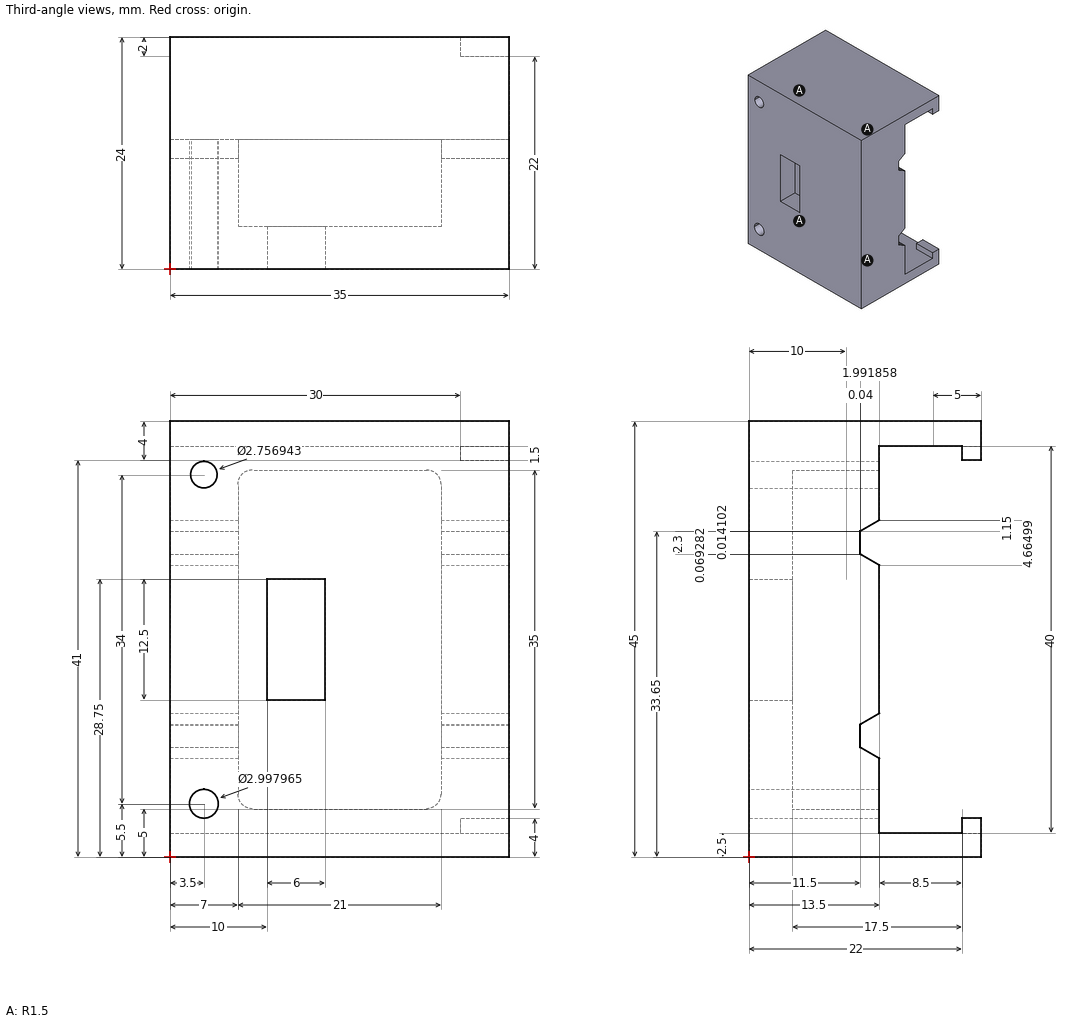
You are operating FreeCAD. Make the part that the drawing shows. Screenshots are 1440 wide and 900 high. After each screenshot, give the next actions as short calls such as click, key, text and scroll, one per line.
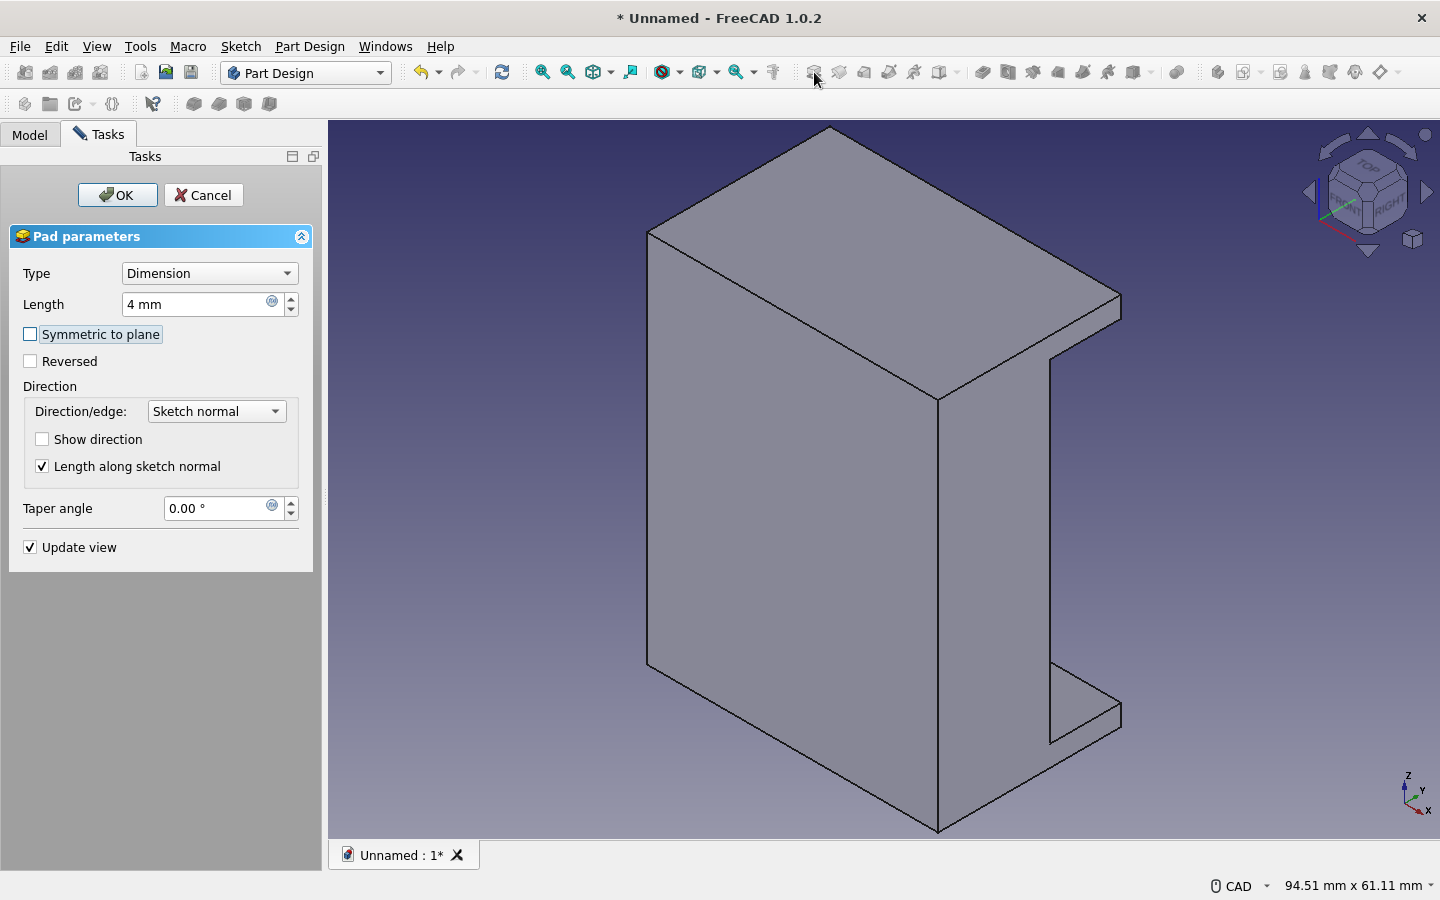
click(31, 361)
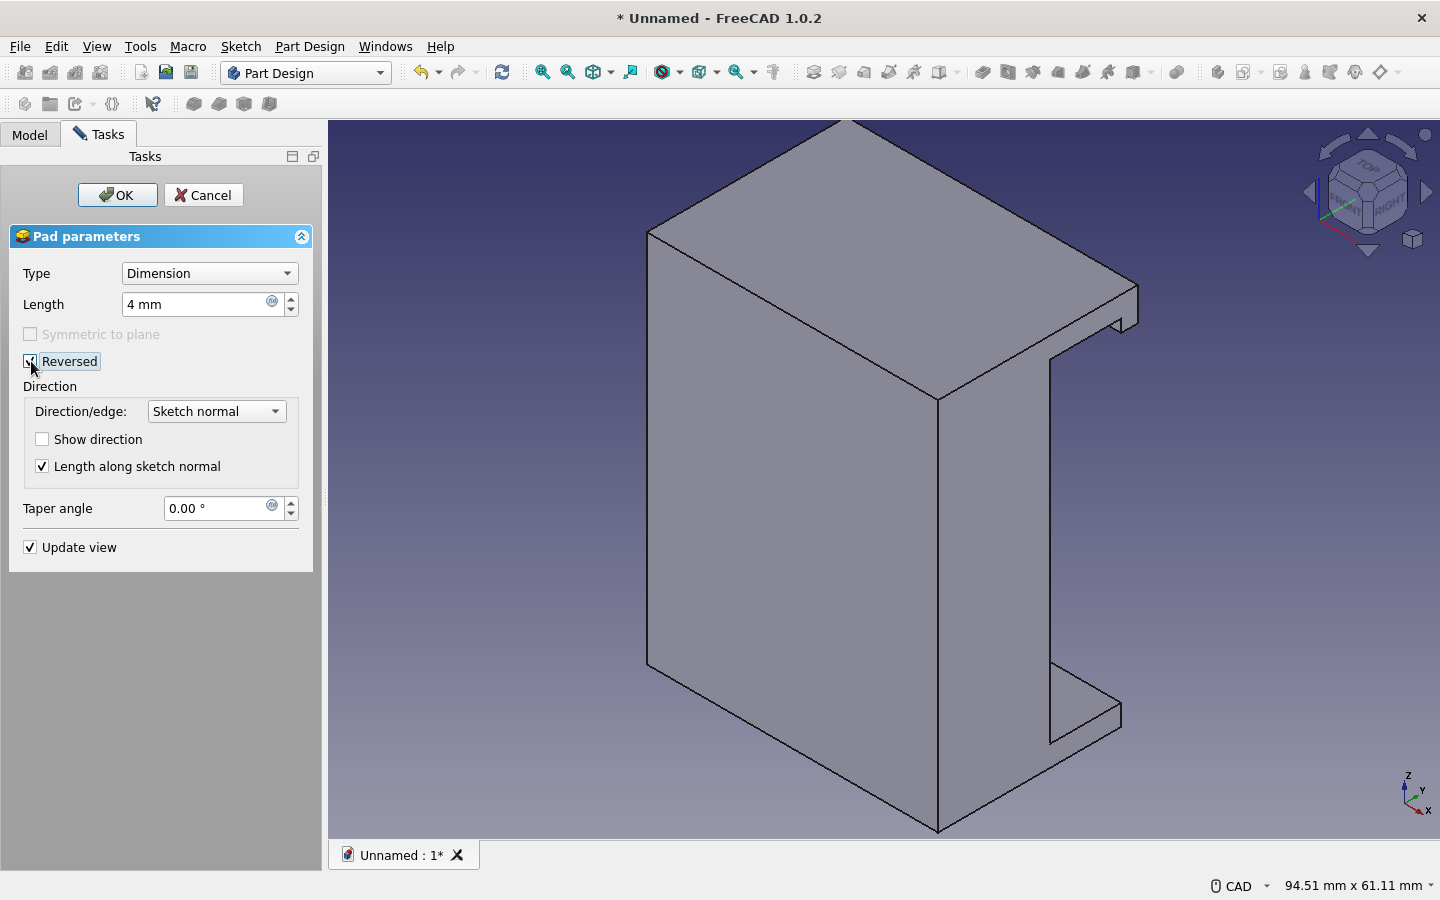
click(118, 195)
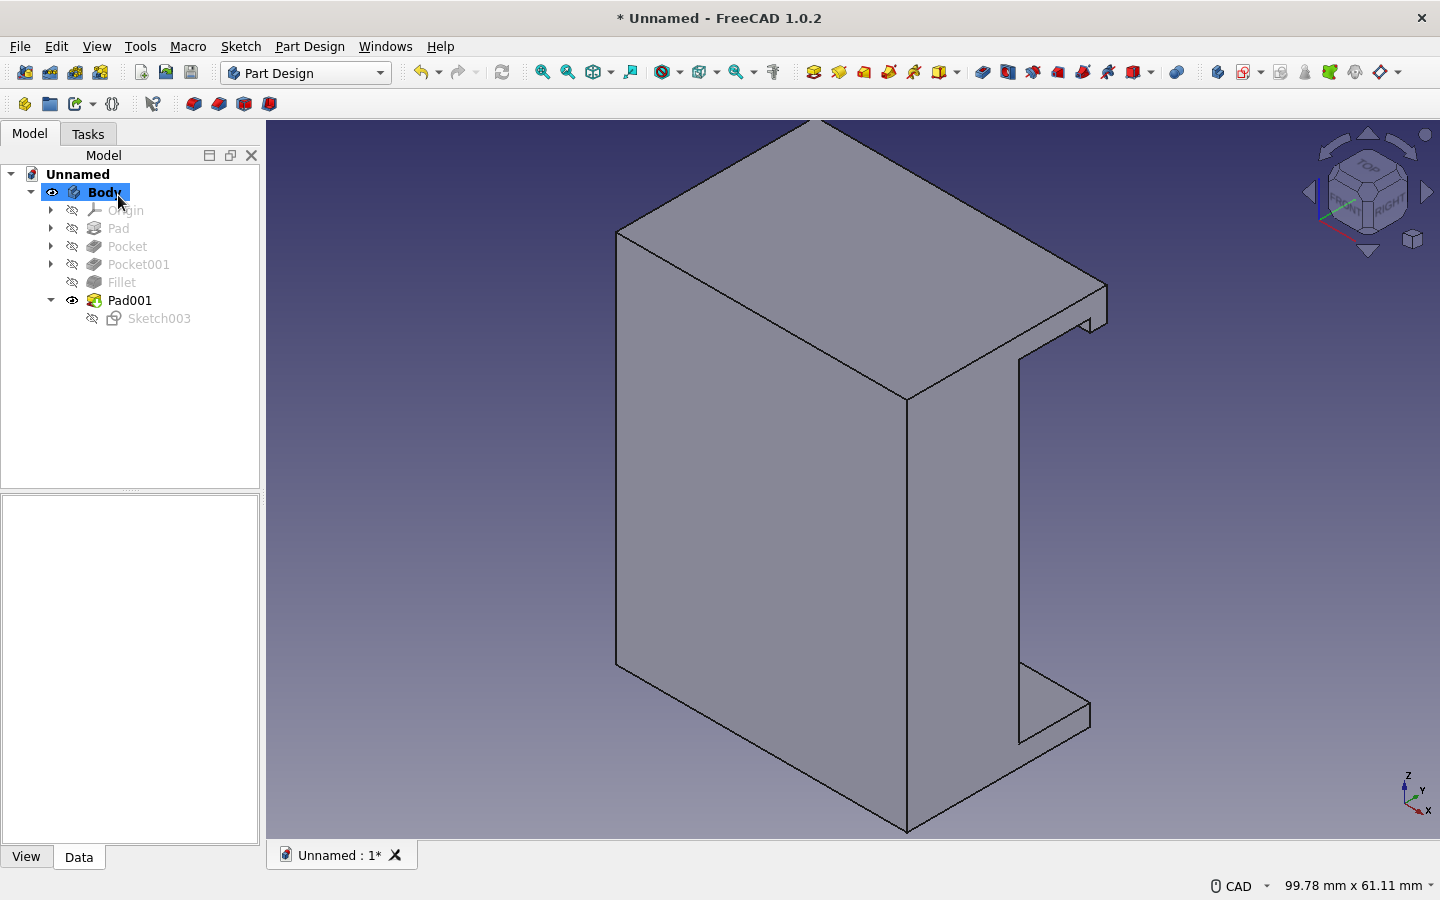
click(543, 72)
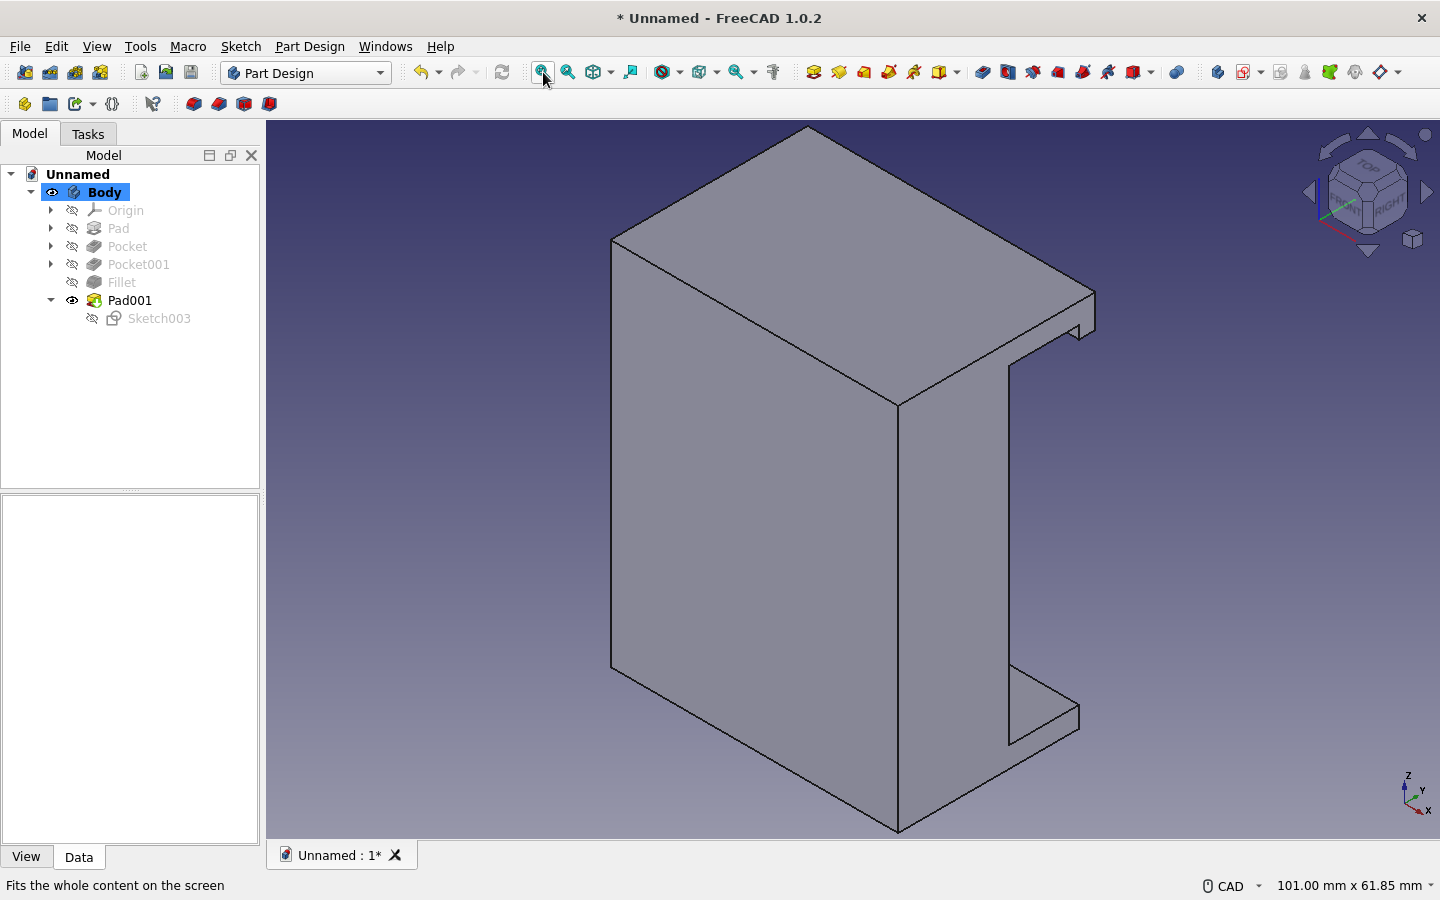
key(5)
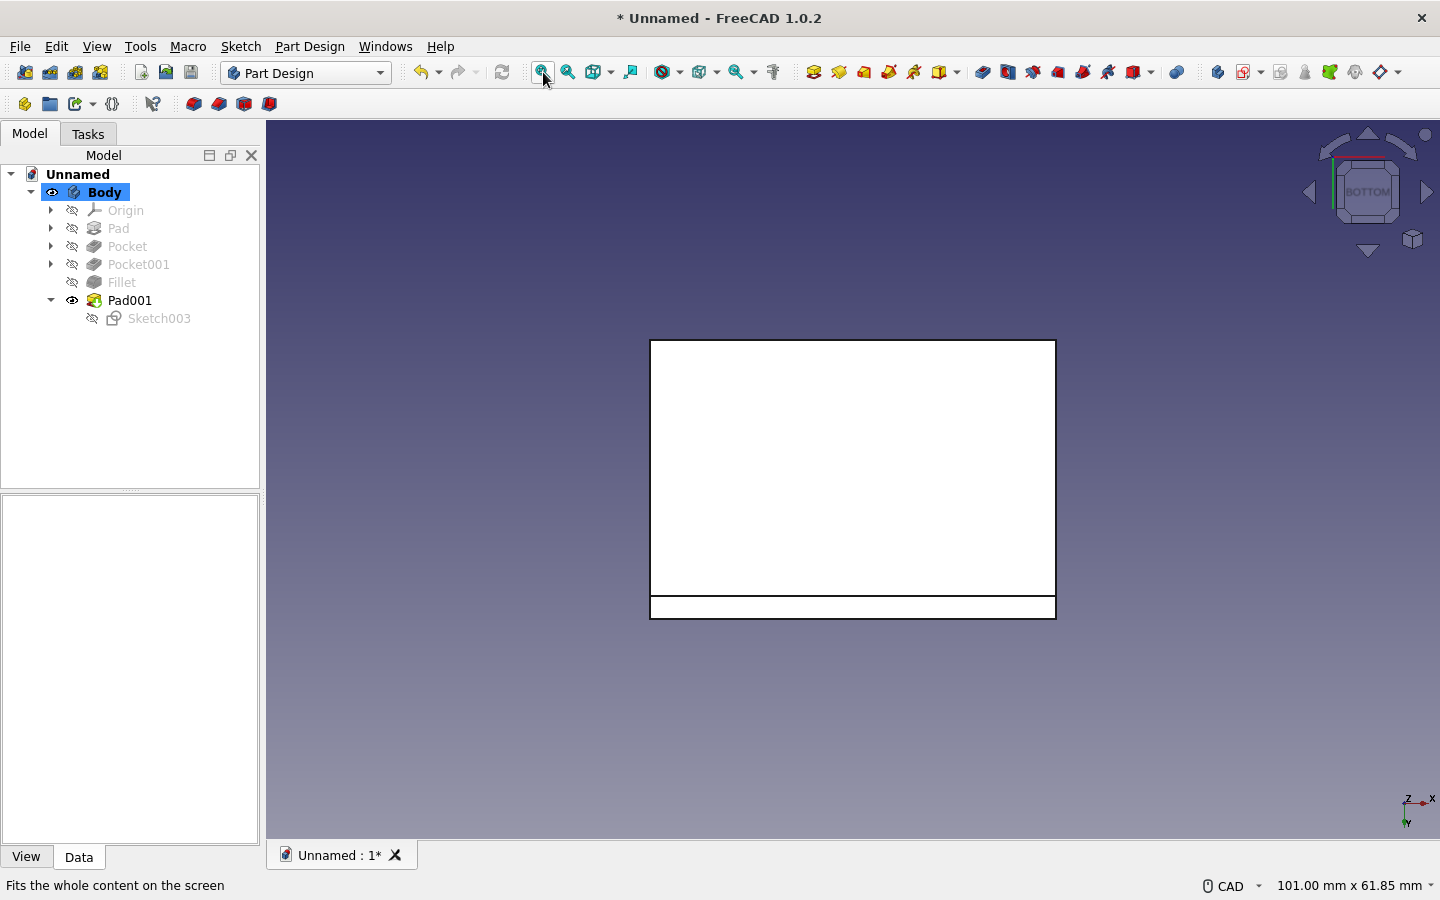
click(543, 72)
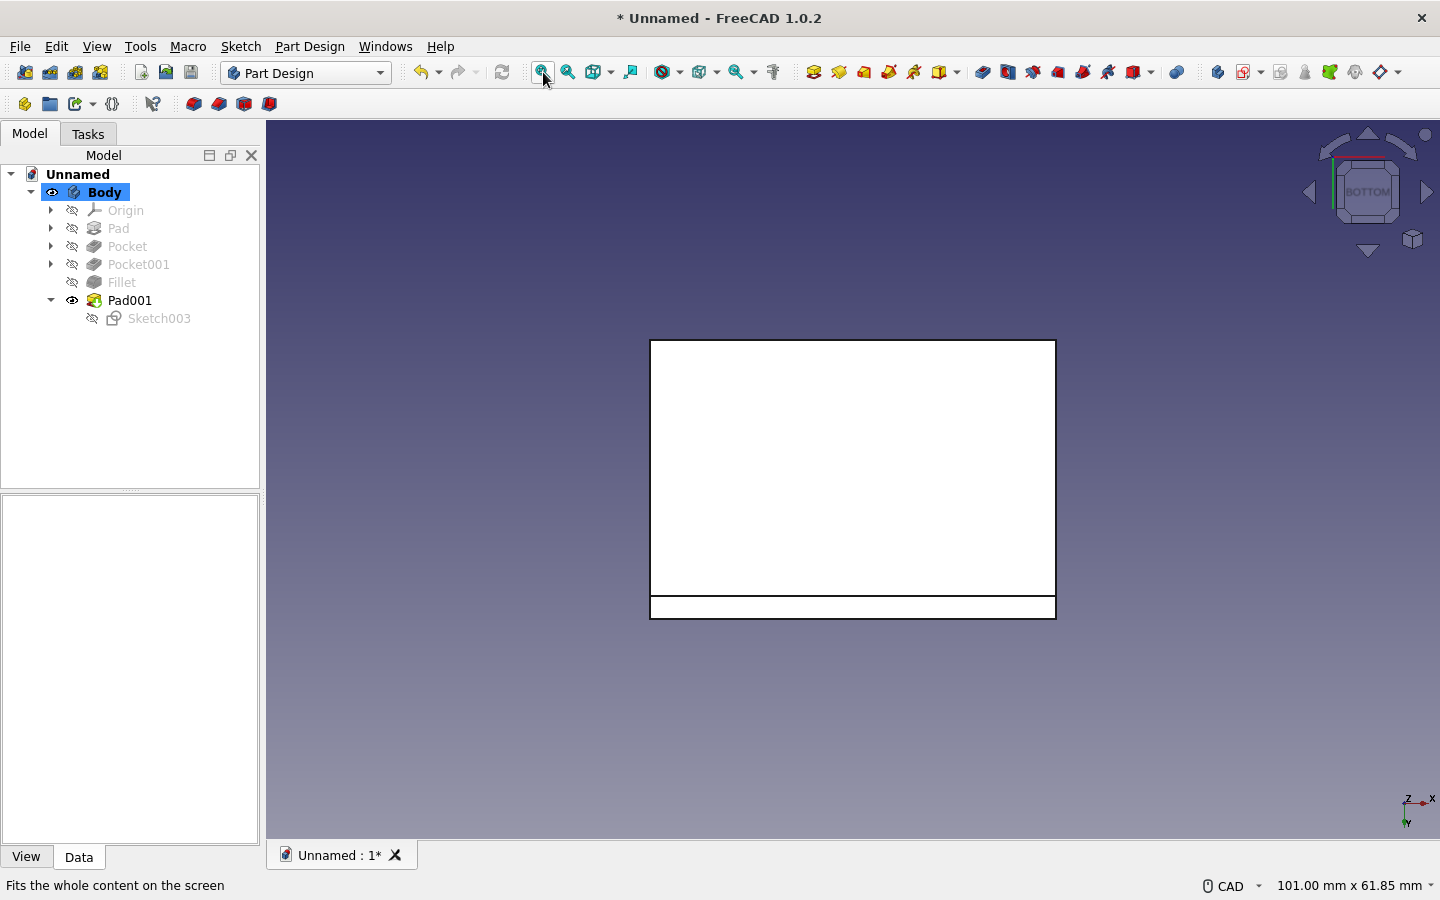
click(911, 467)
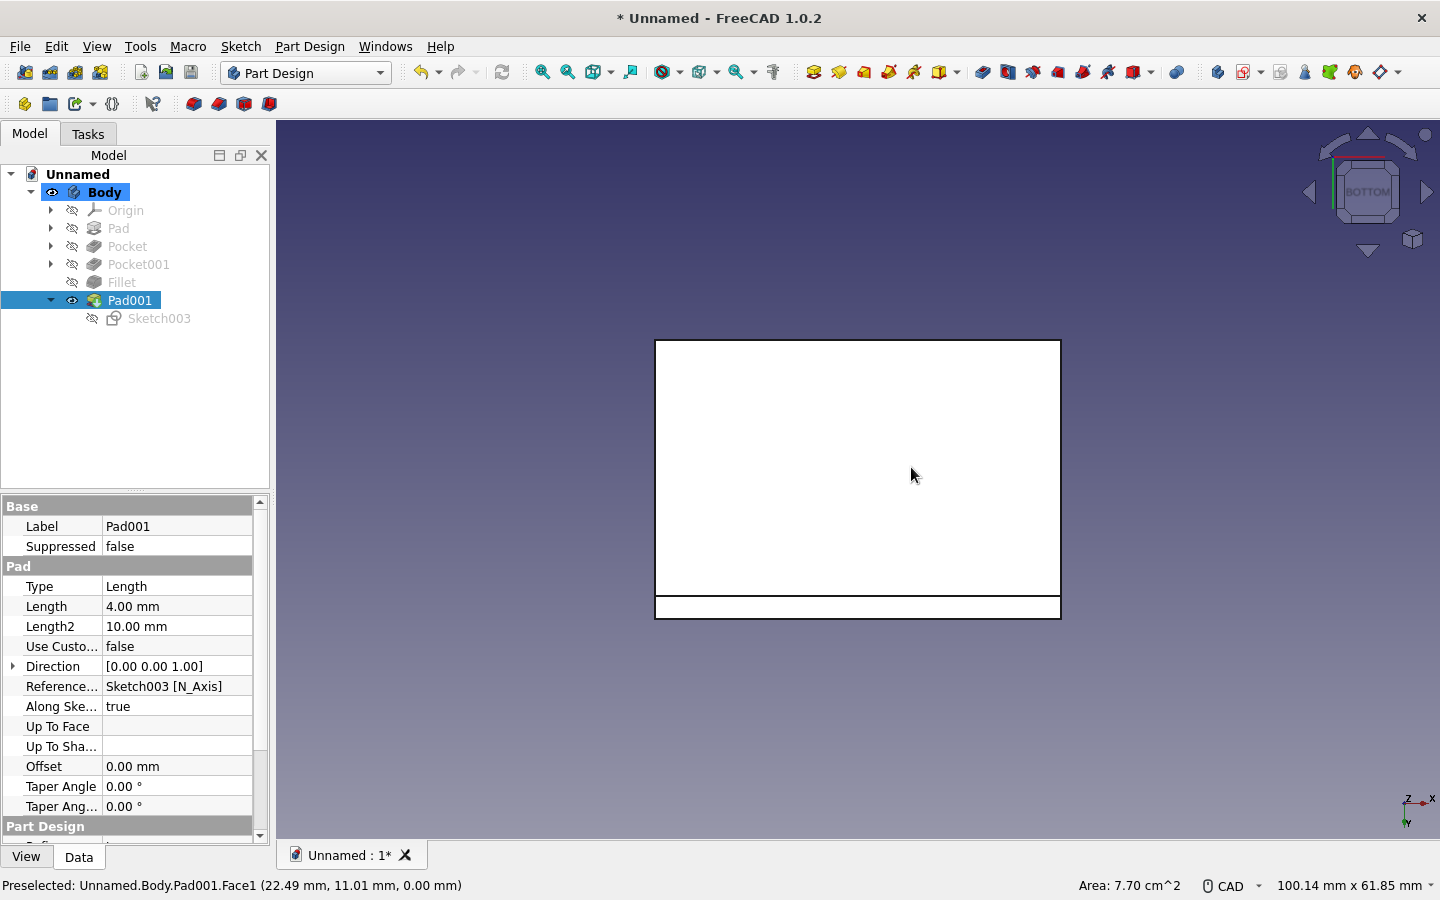
click(1242, 72)